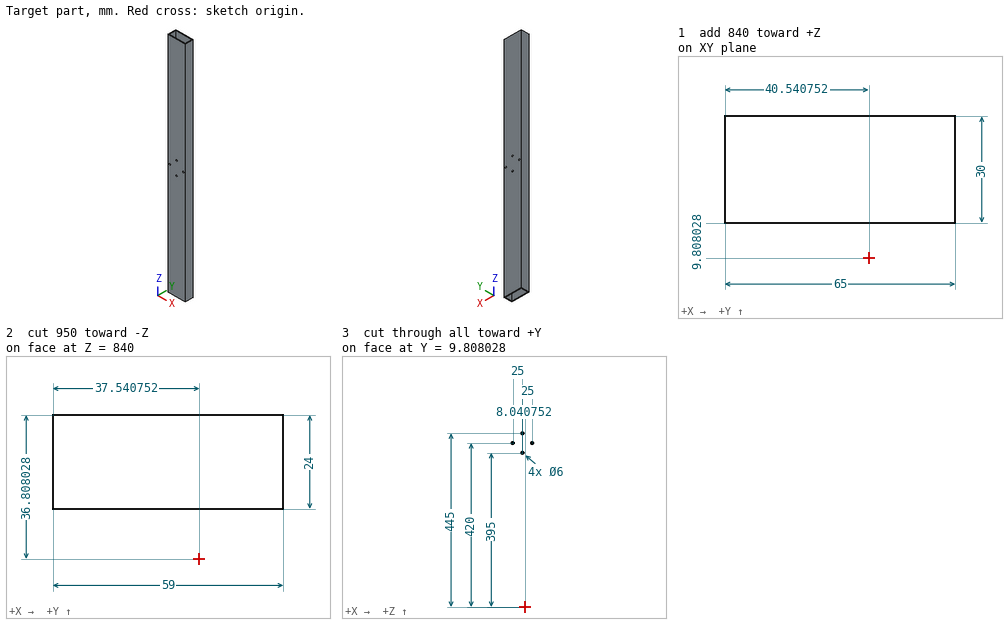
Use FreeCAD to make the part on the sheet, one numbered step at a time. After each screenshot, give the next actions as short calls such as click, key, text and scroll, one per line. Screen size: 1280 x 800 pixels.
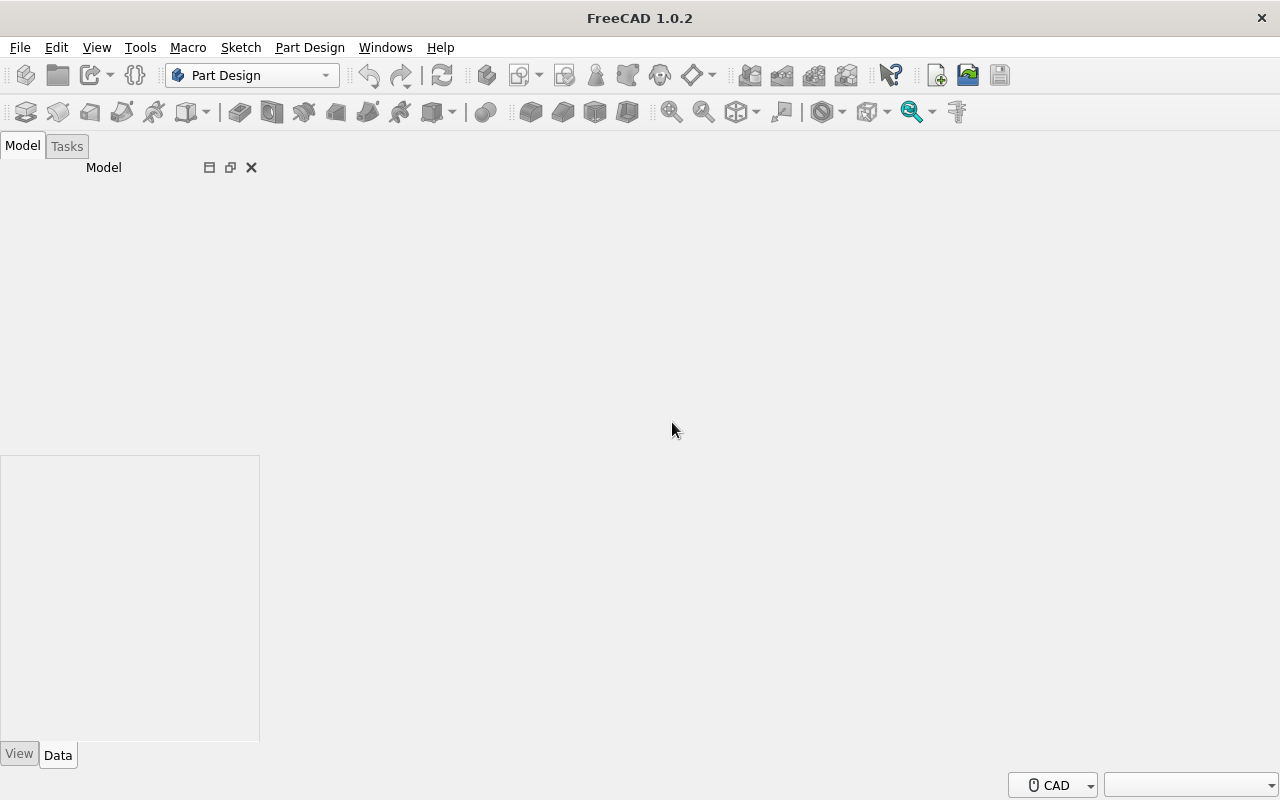
click(936, 76)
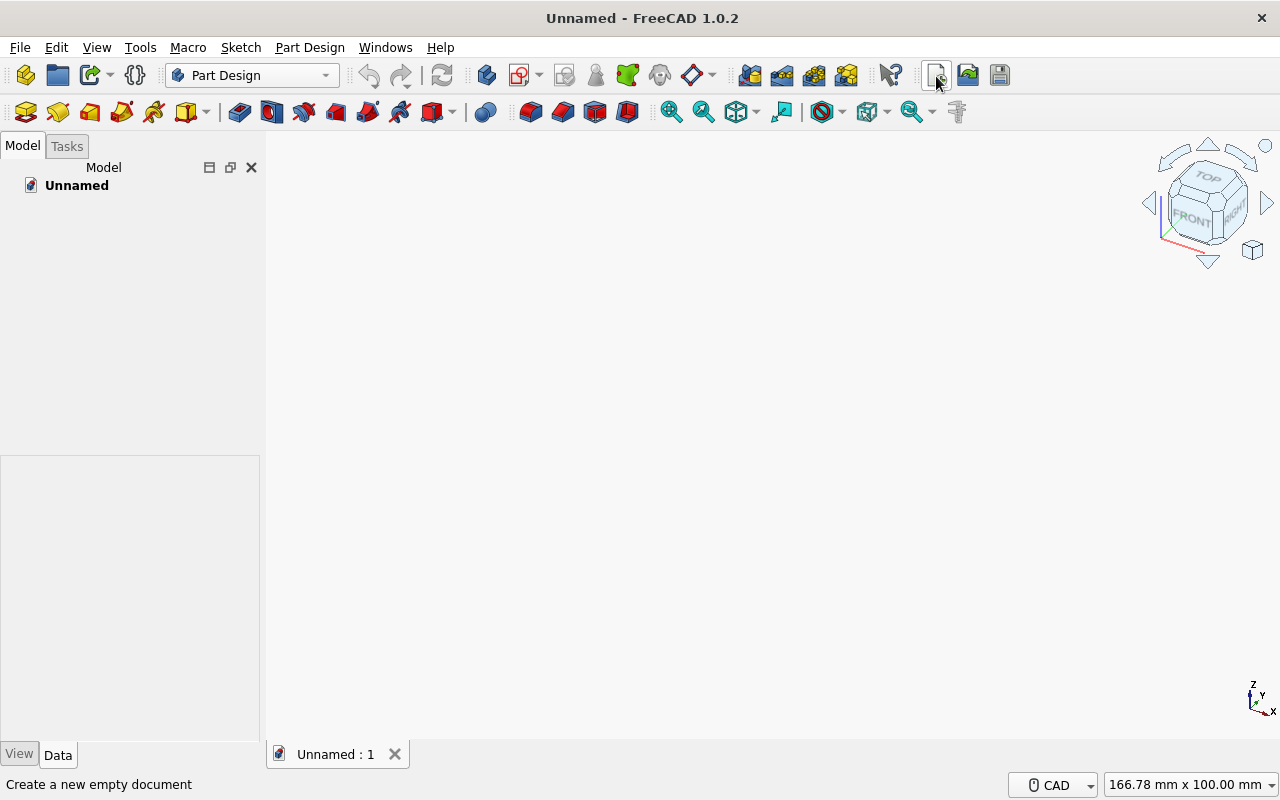
click(520, 76)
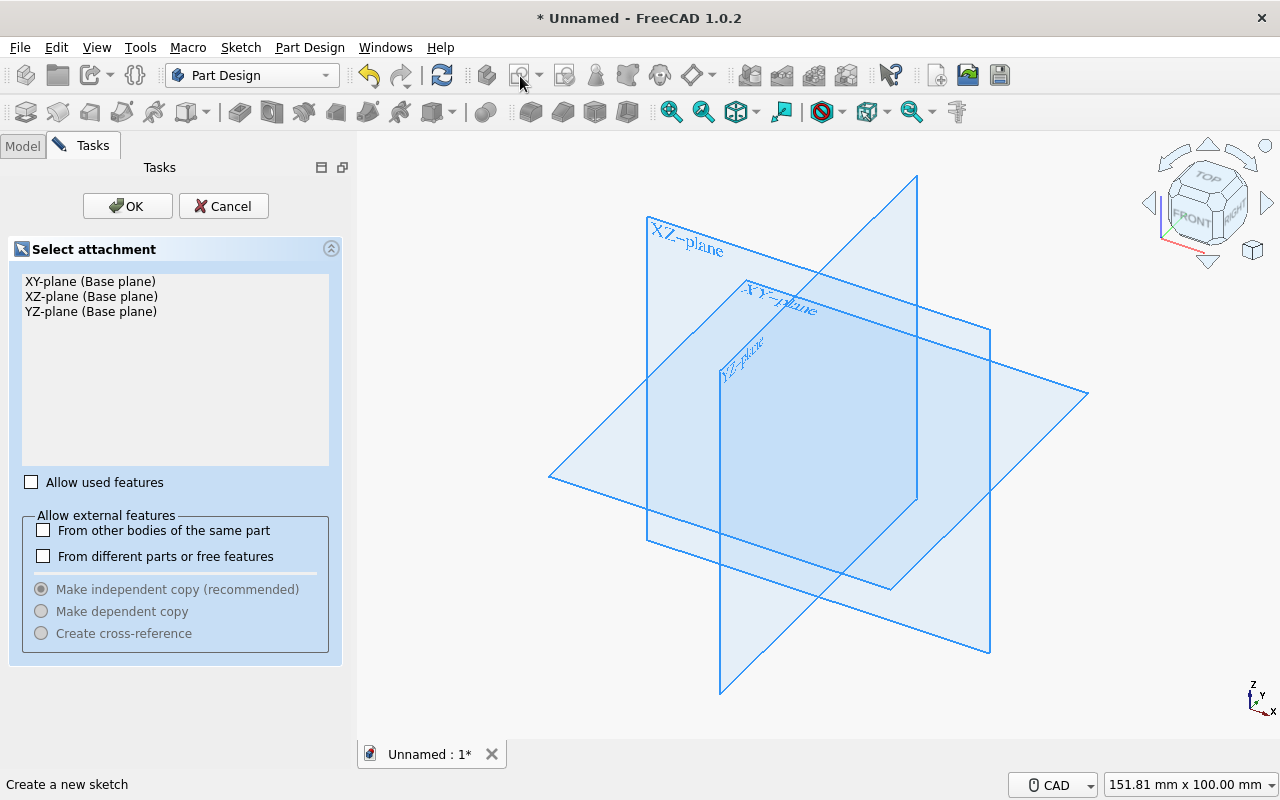
click(82, 282)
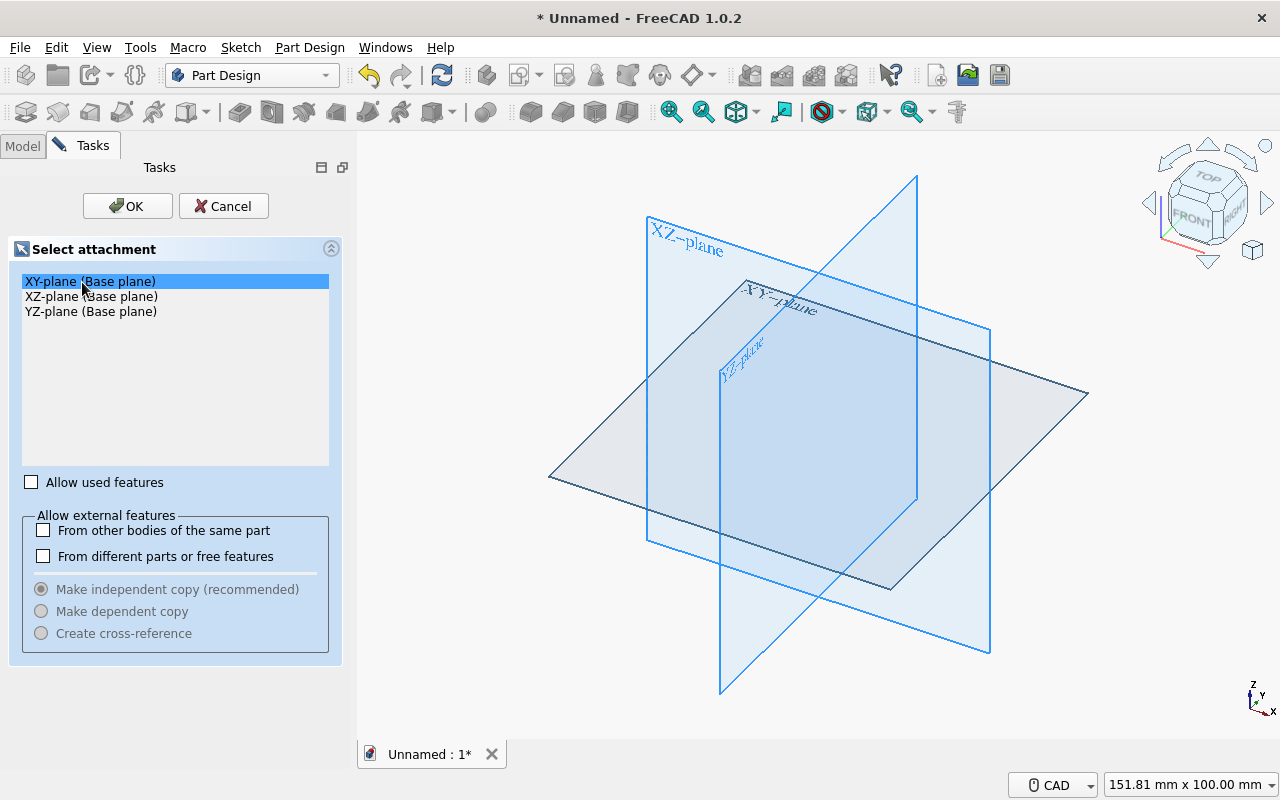
click(128, 206)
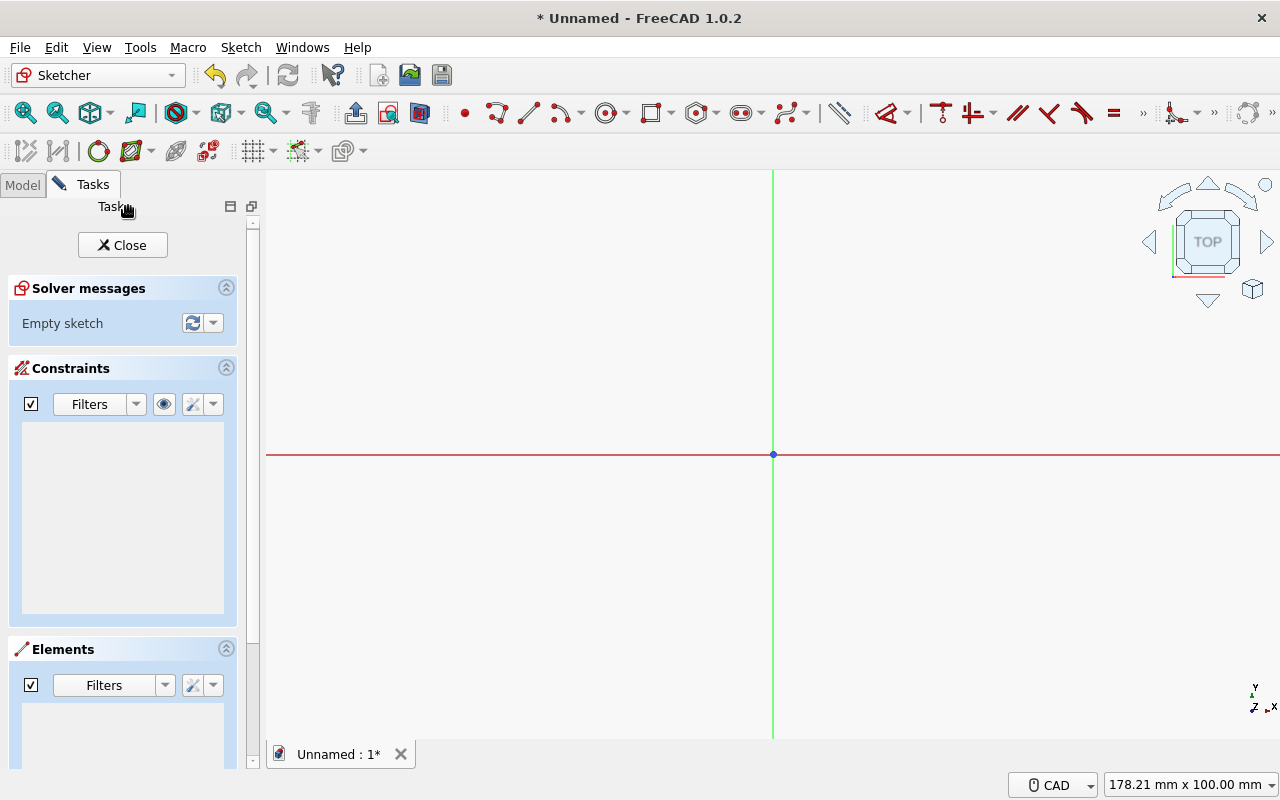
scroll(774, 198, up, 2)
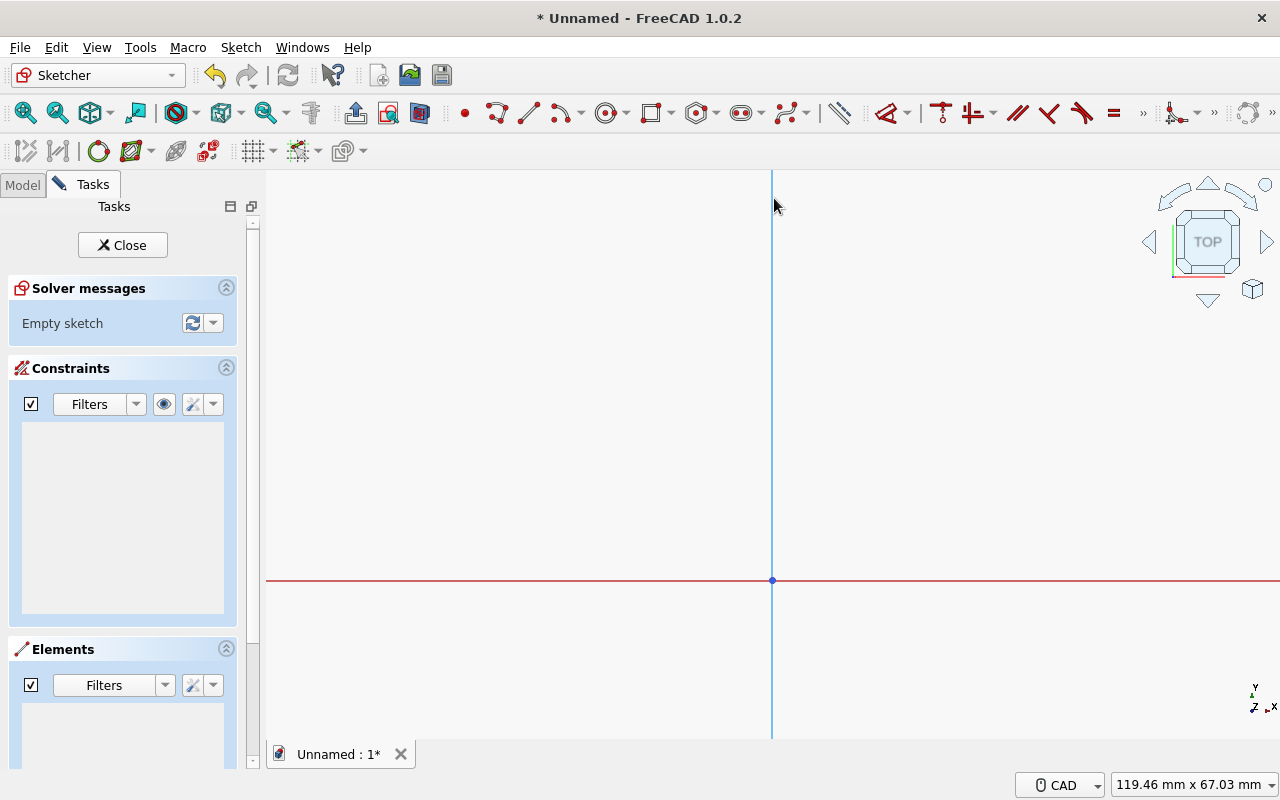
click(652, 114)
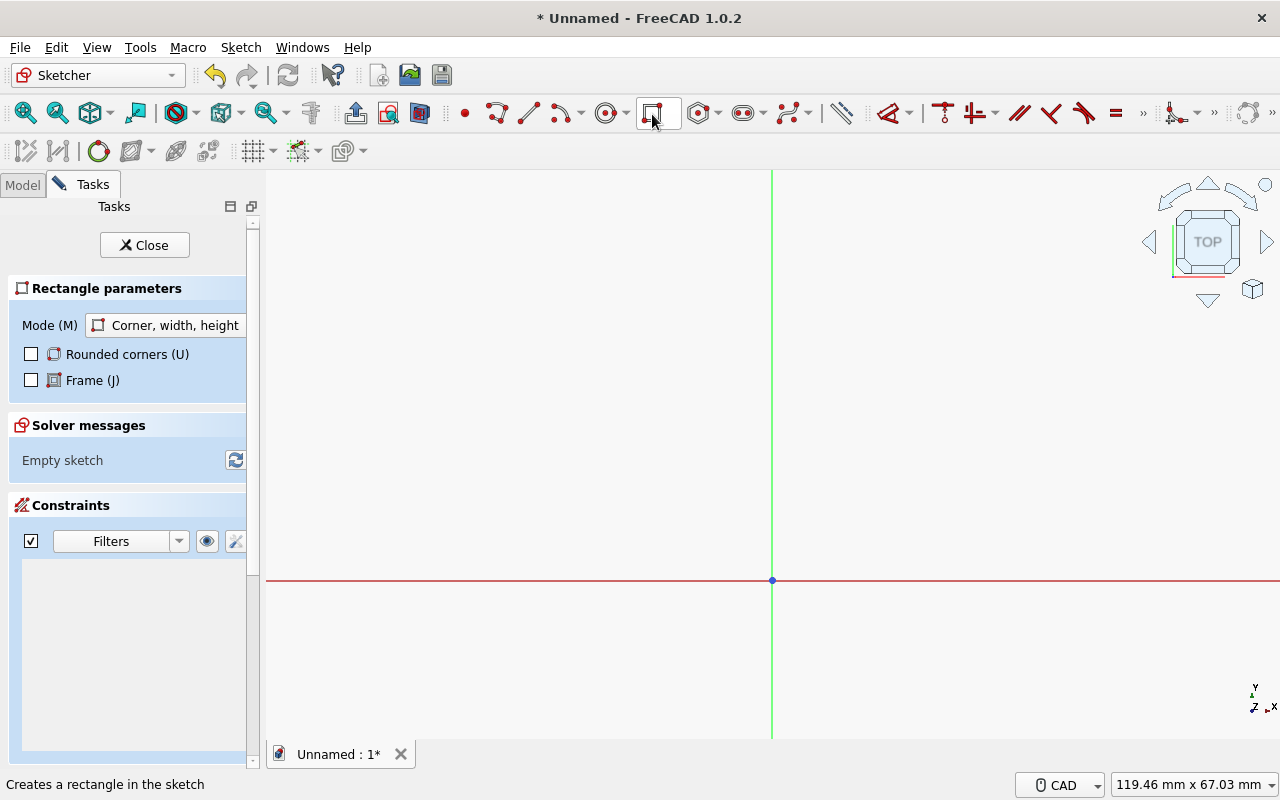
click(428, 243)
move(980, 497)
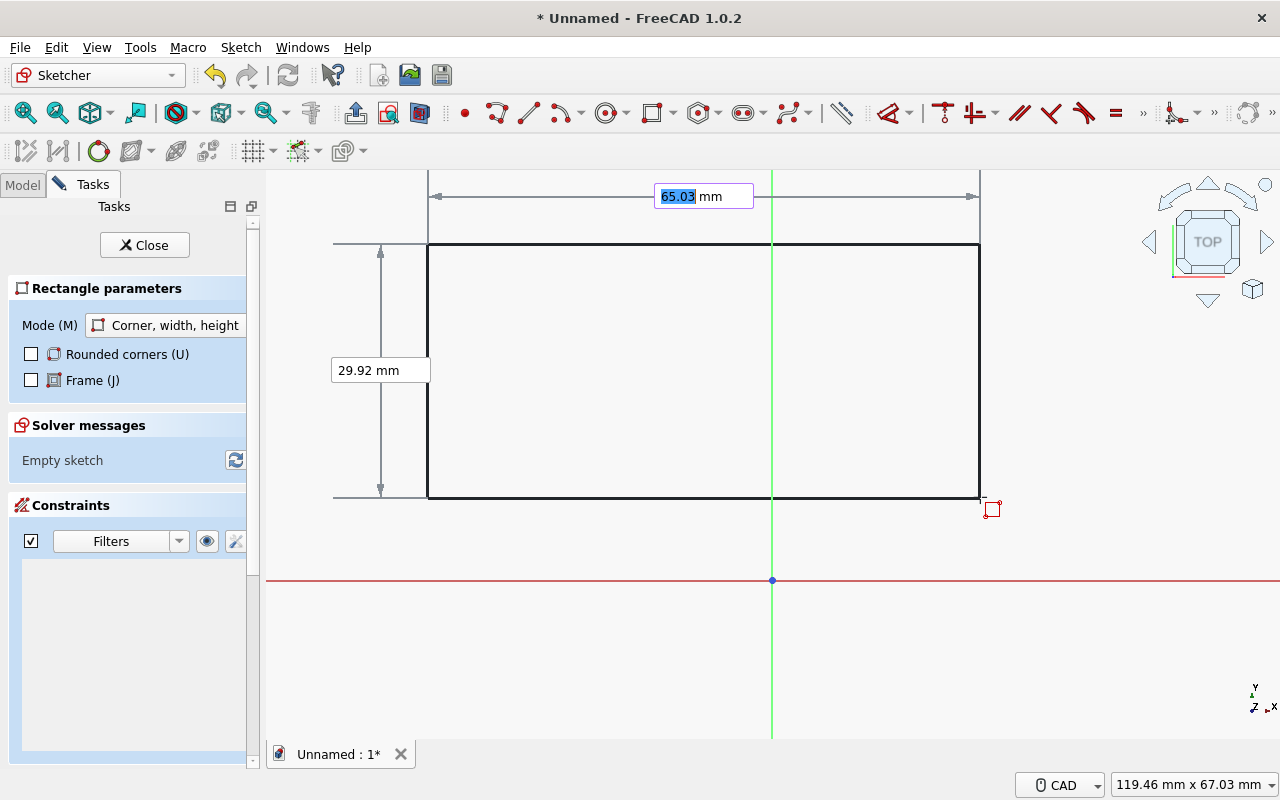
text(65)
key(Tab)
text(30)
key(Return)
key(Escape)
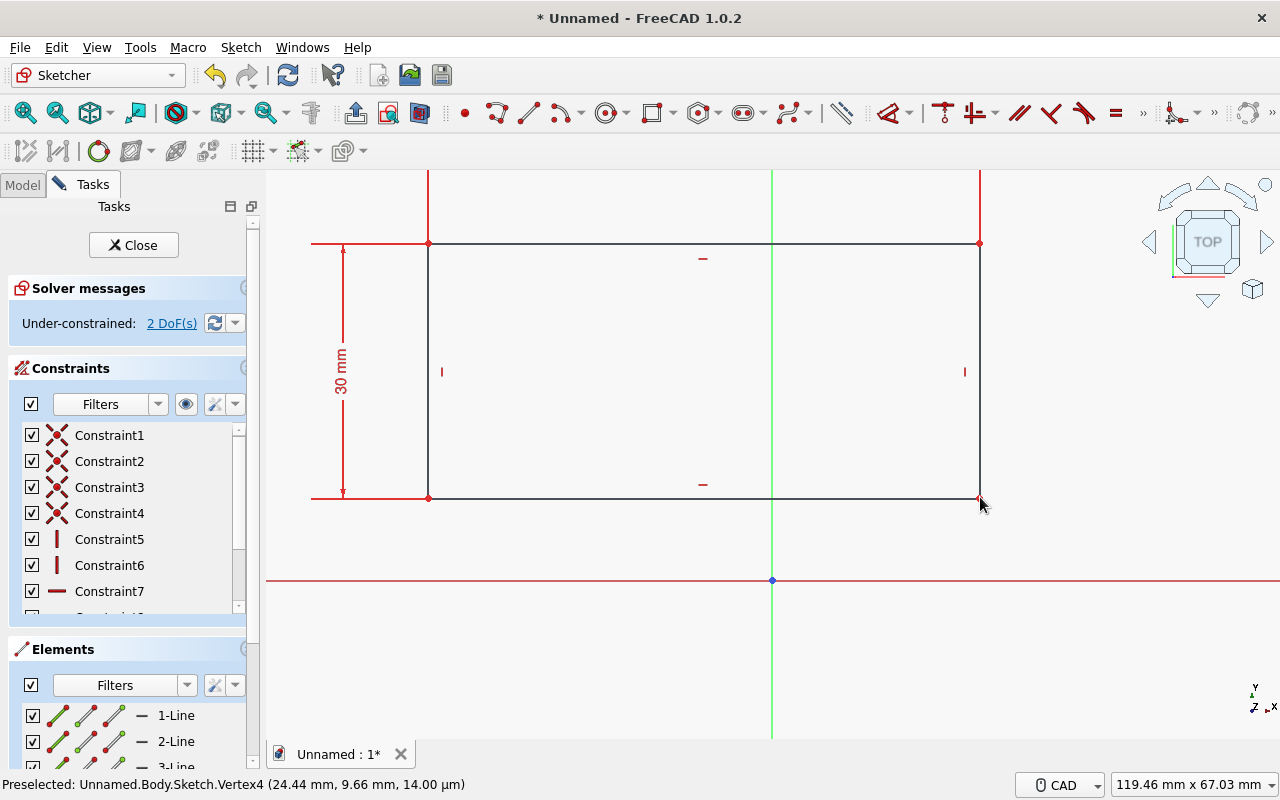
click(888, 114)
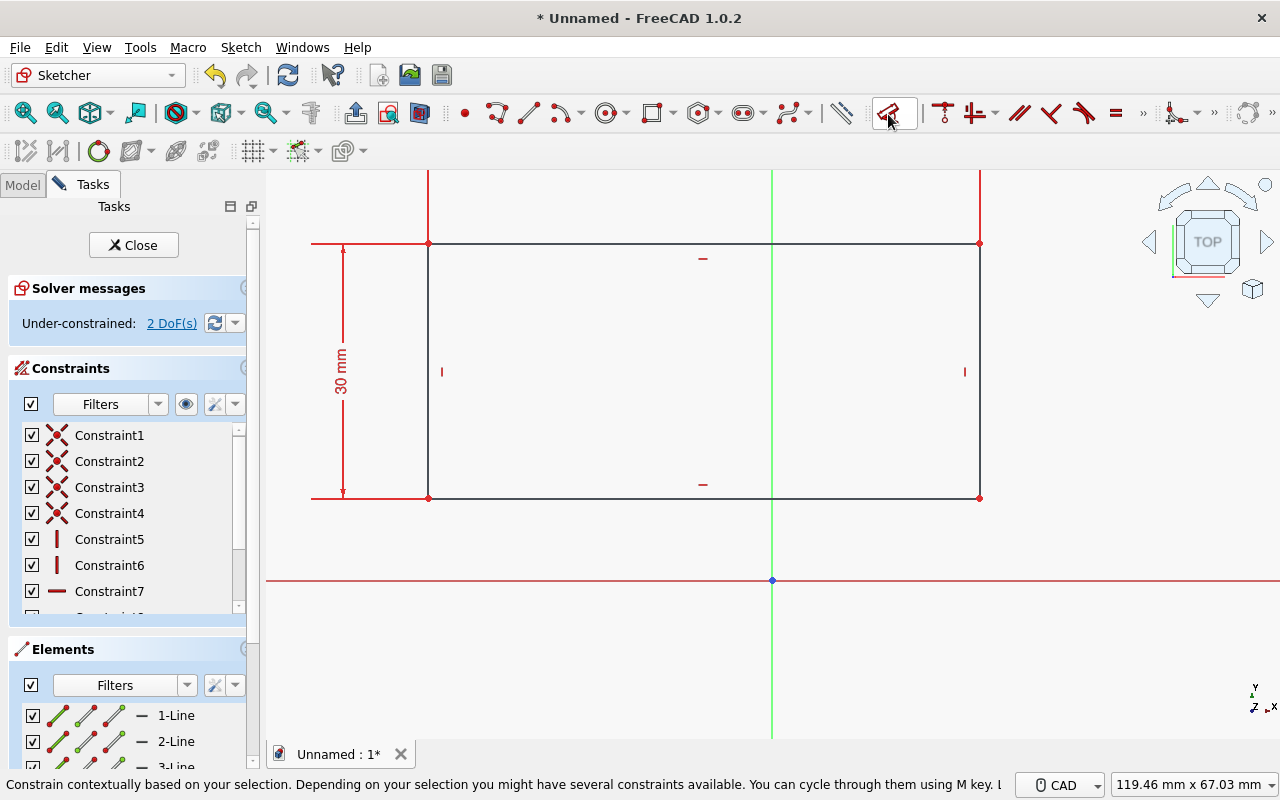
click(428, 499)
click(394, 540)